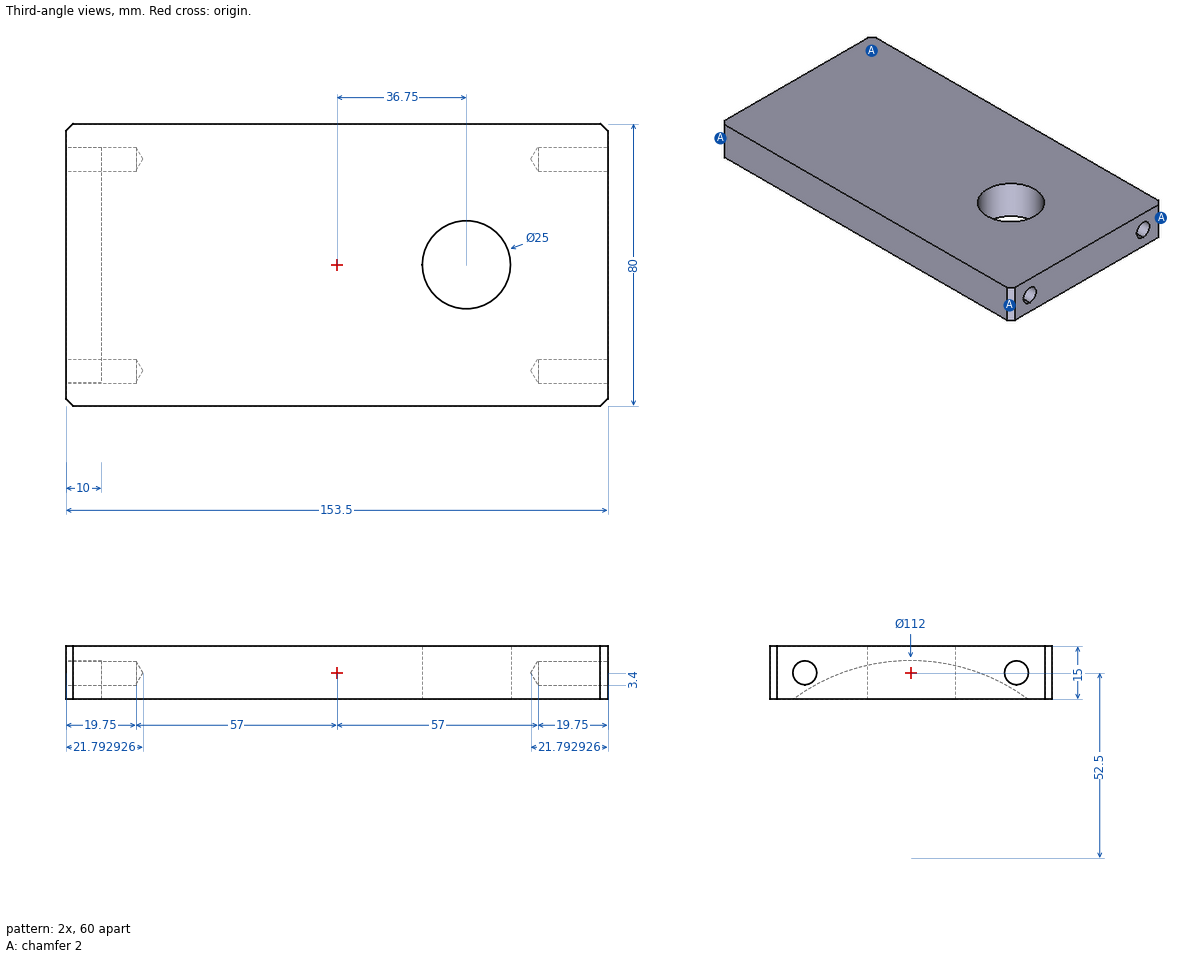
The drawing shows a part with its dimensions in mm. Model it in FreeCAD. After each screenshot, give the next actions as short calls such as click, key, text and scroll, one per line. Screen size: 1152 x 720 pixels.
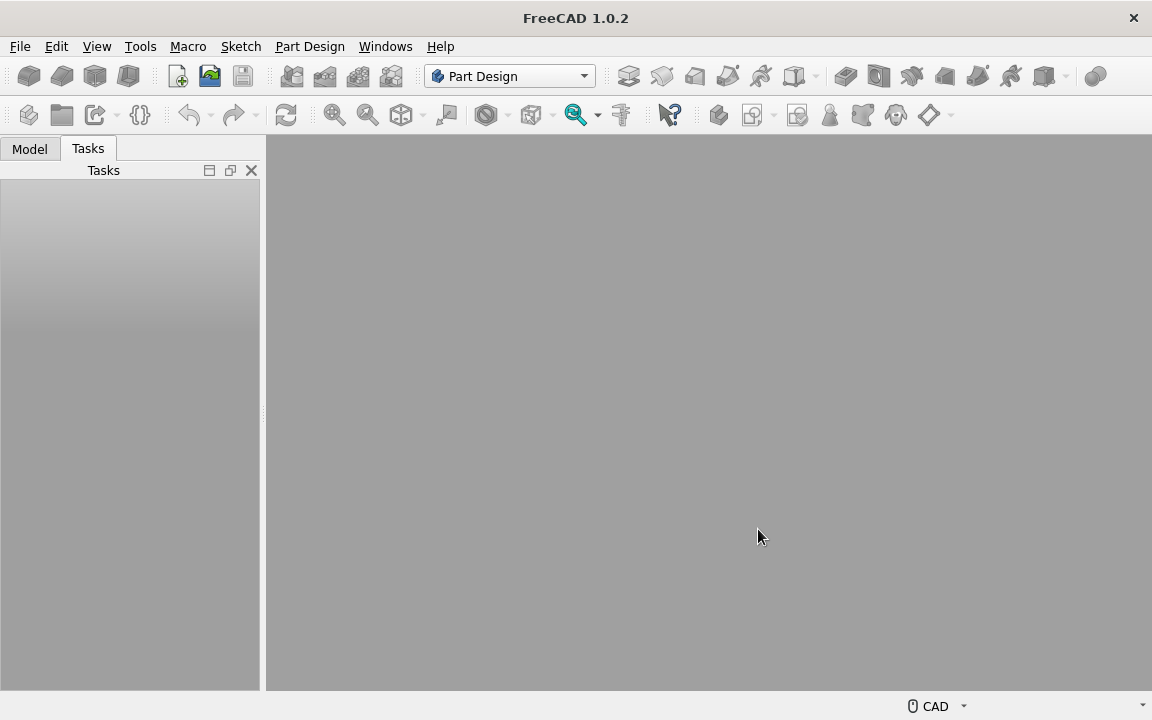
click(177, 76)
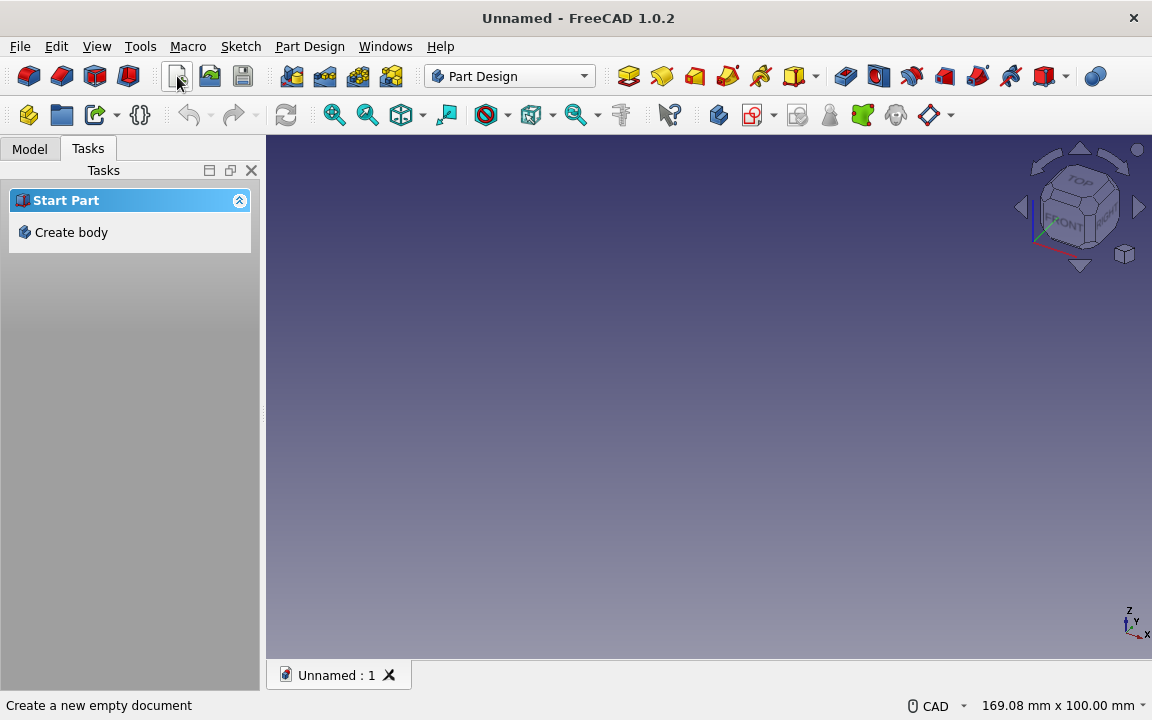
click(752, 116)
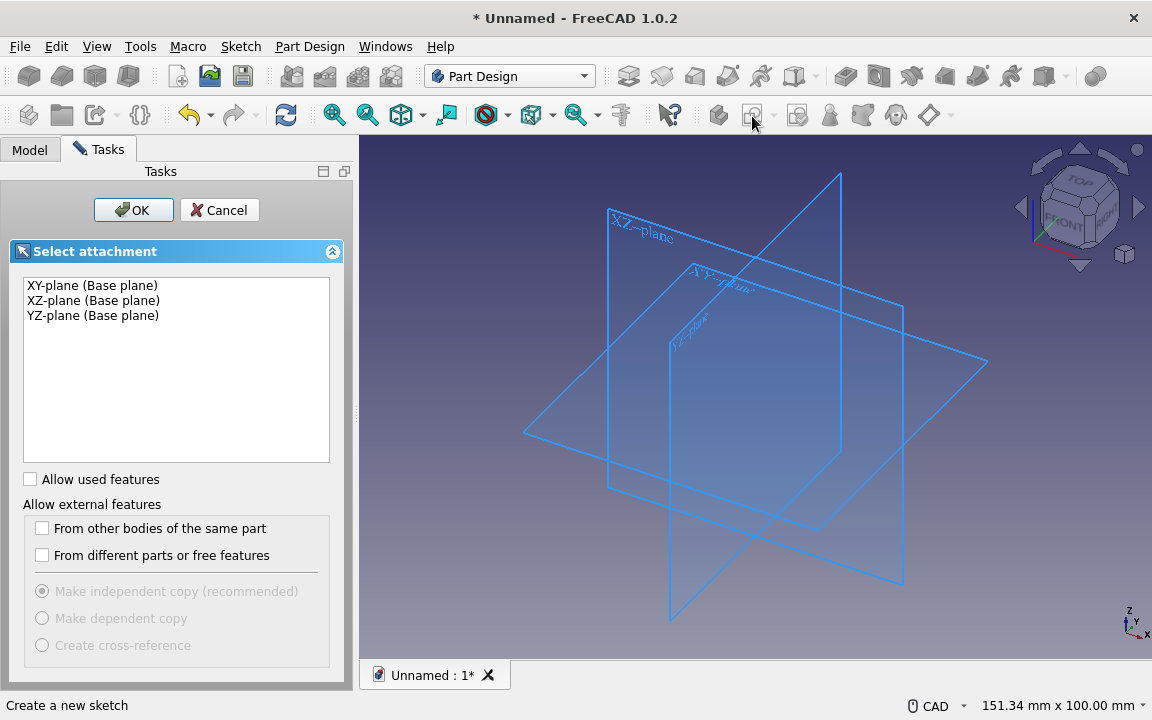
click(84, 286)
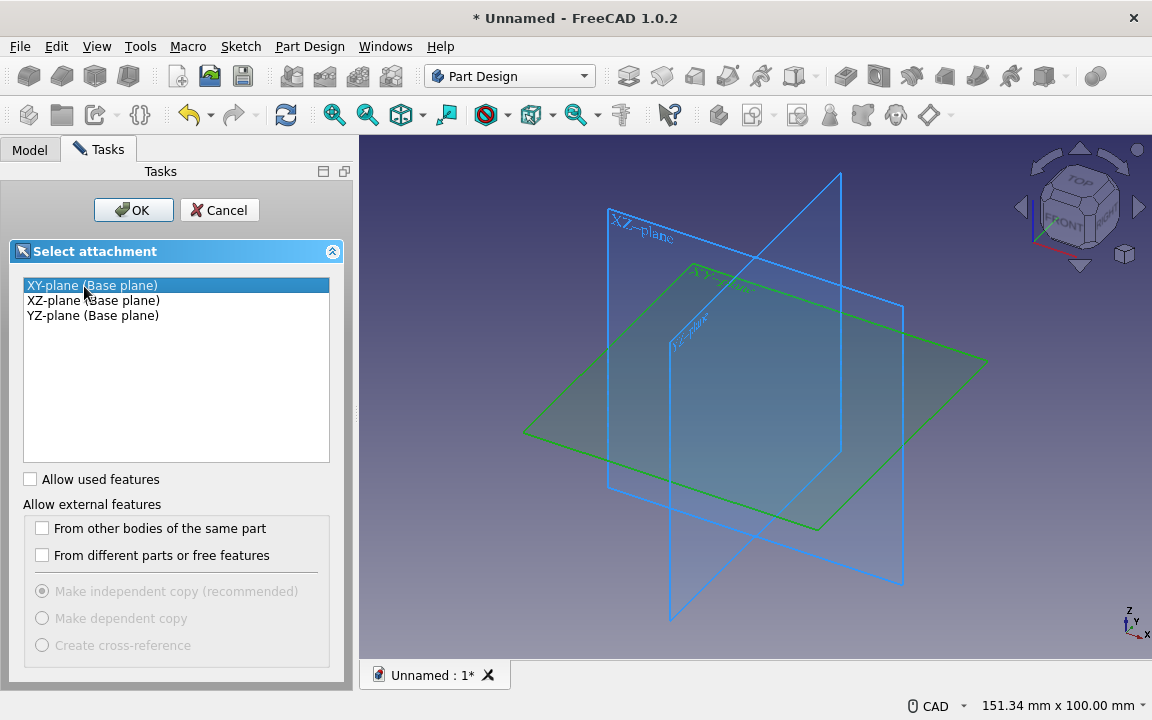
click(134, 210)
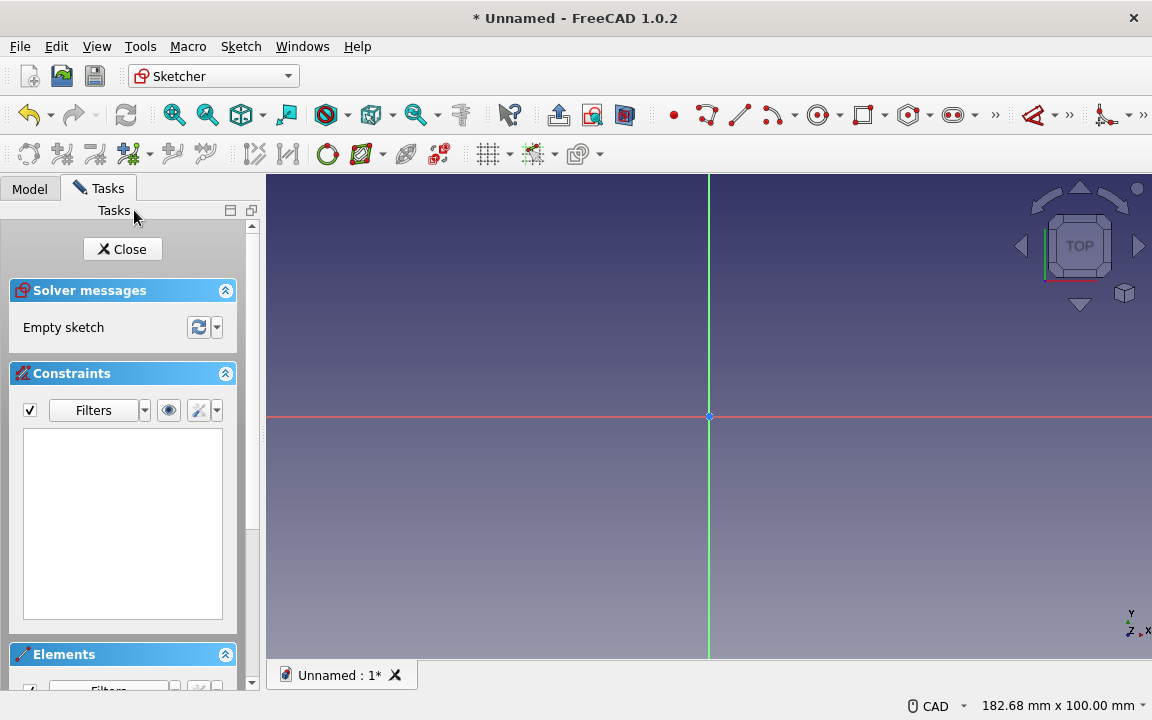
scroll(501, 416, down, 2)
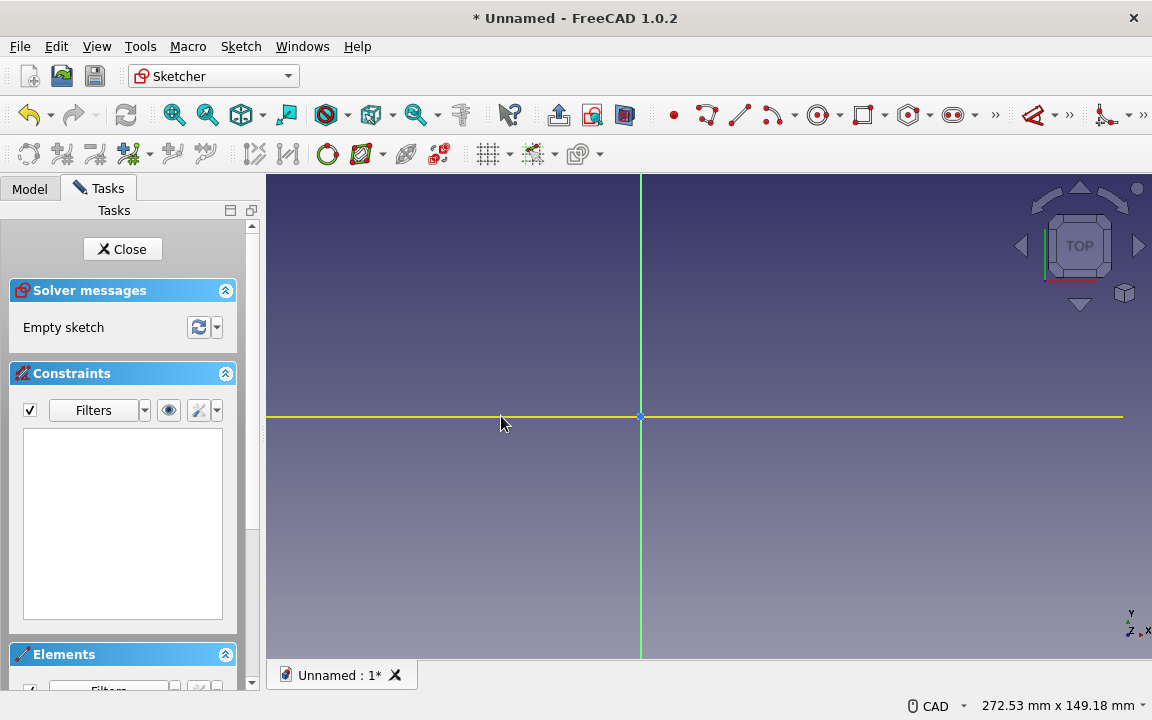
key(g)
key(v)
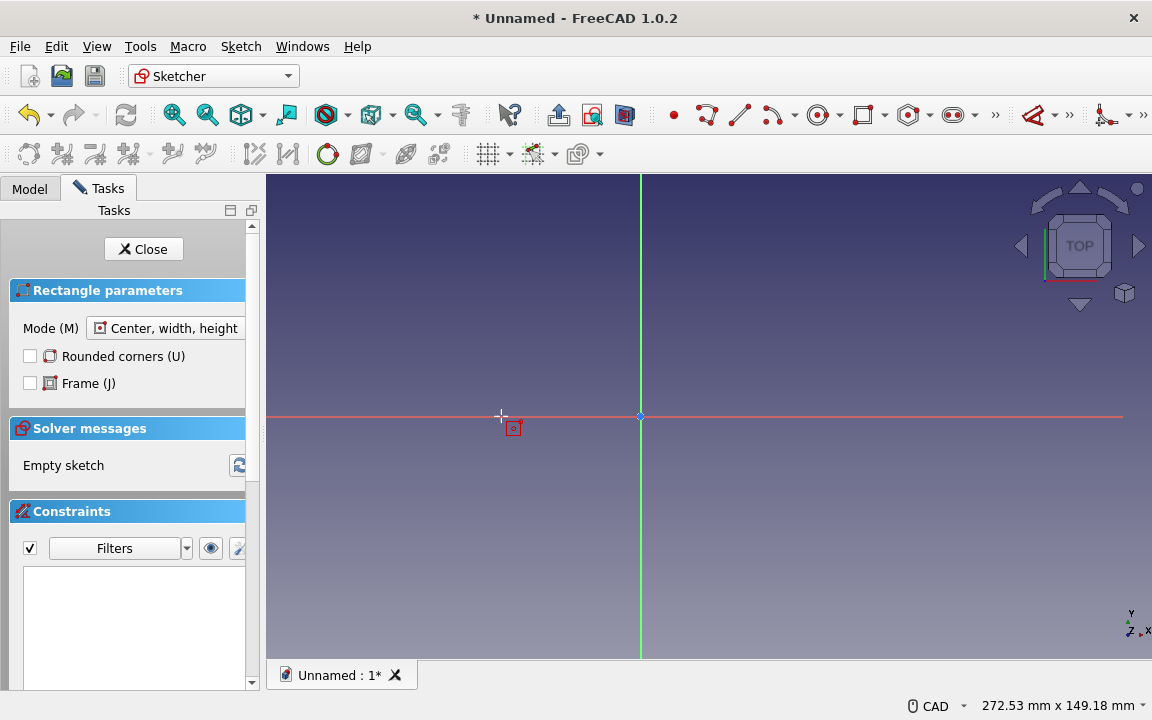
click(641, 416)
move(890, 286)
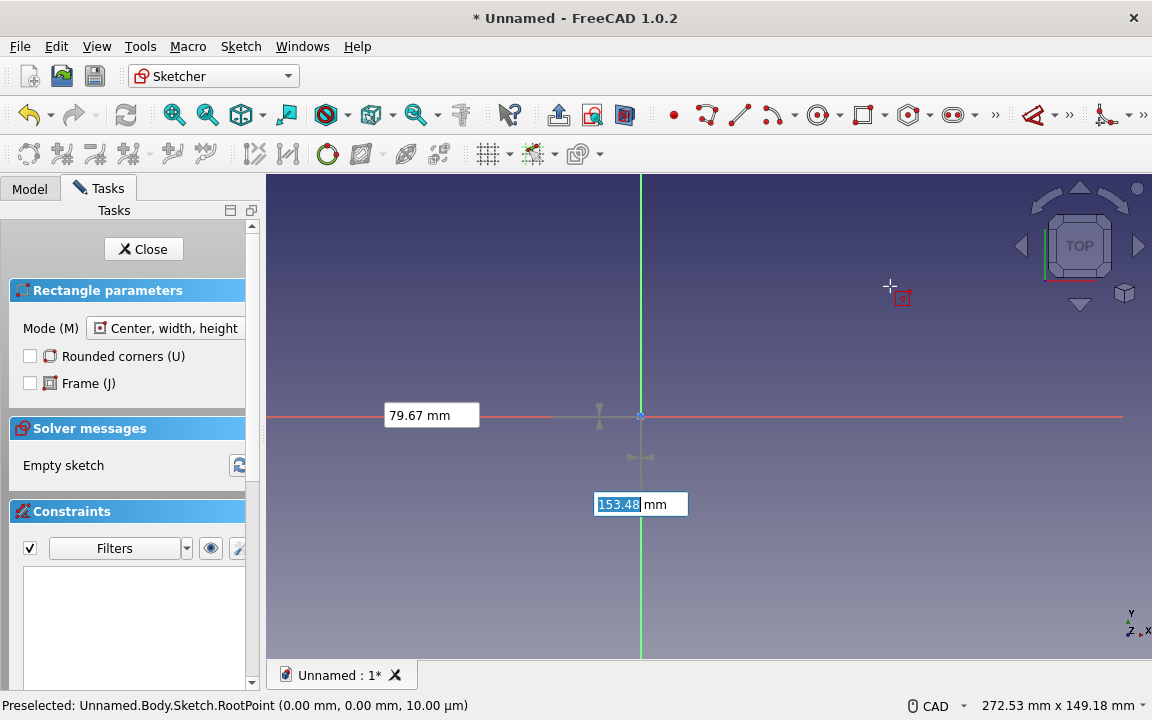
text(153.5)
key(Tab)
text(80)
key(Return)
key(Escape)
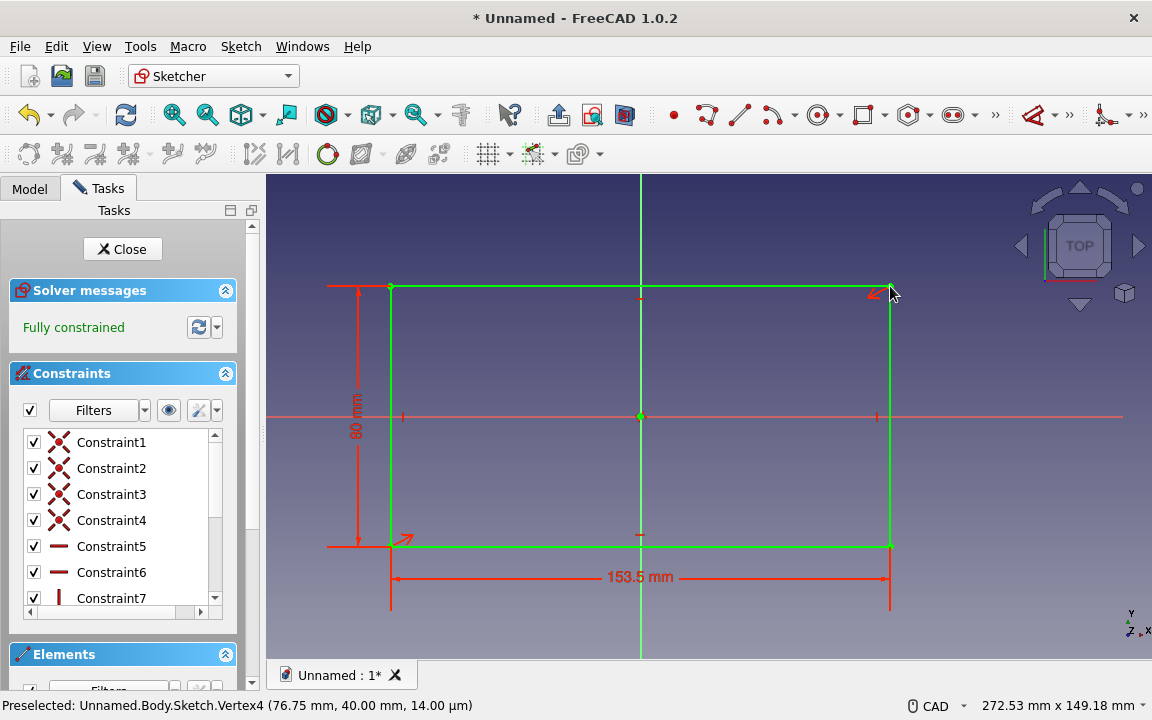
click(123, 249)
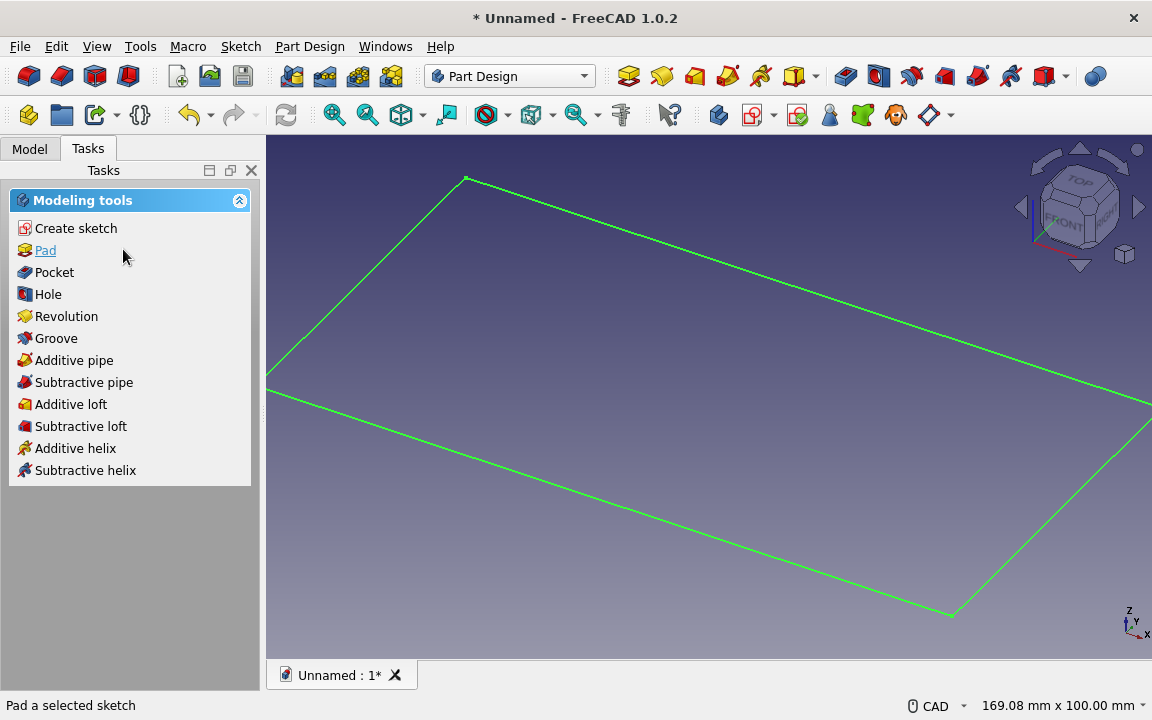
click(629, 76)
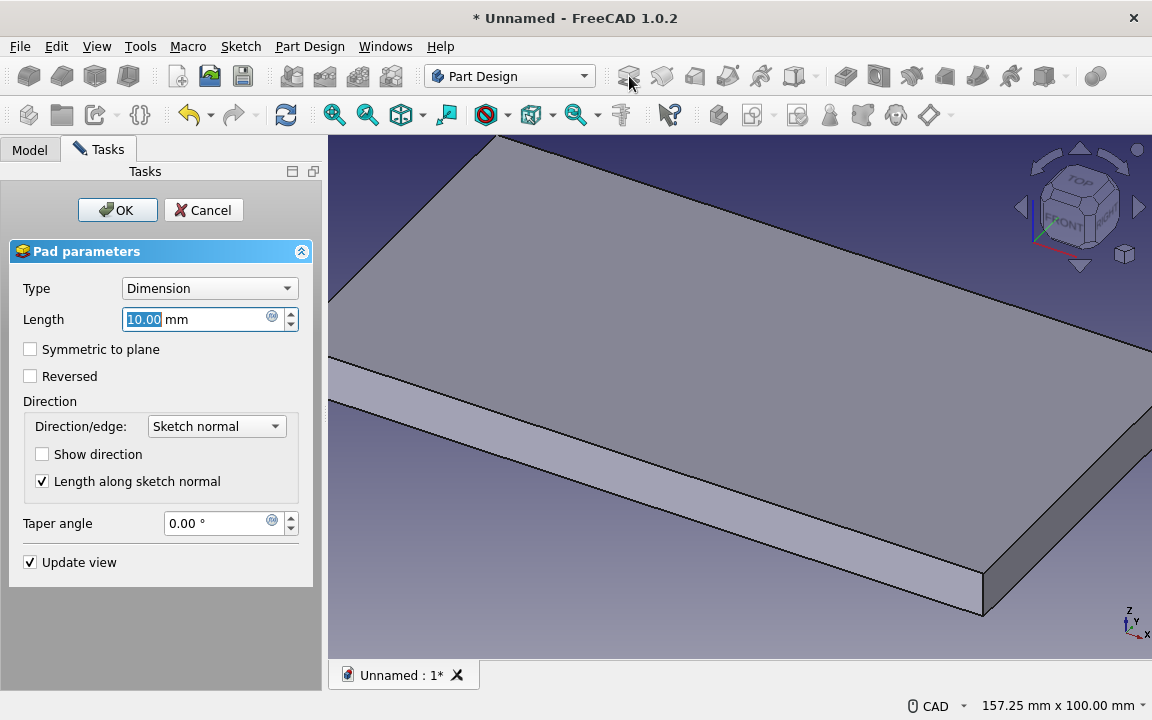
text(15)
key(Tab)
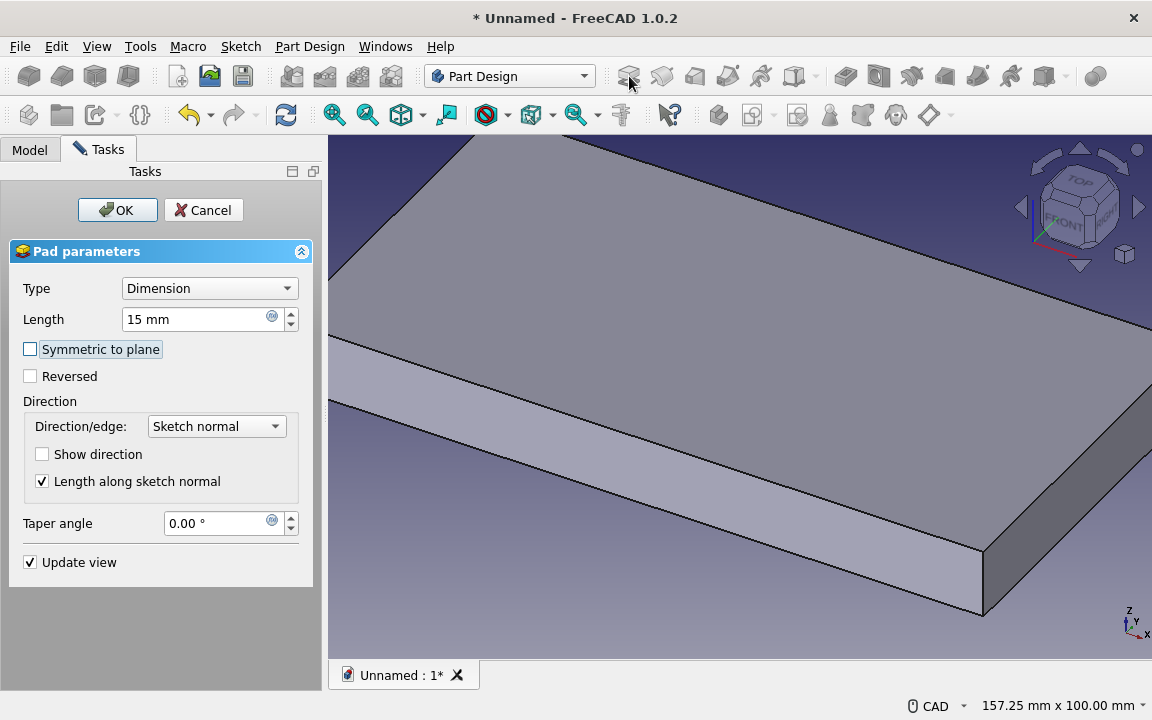
click(31, 349)